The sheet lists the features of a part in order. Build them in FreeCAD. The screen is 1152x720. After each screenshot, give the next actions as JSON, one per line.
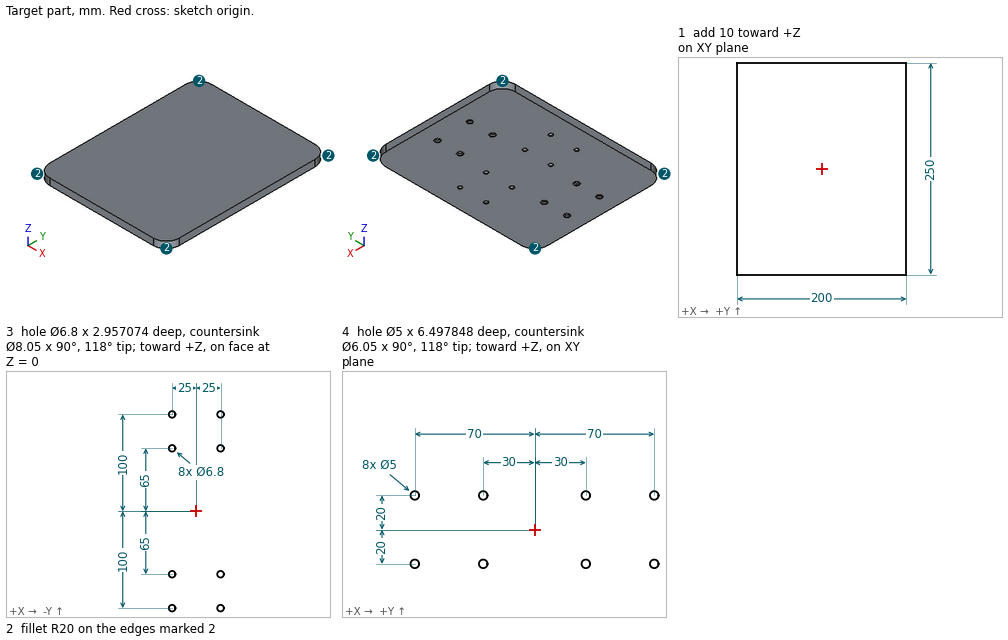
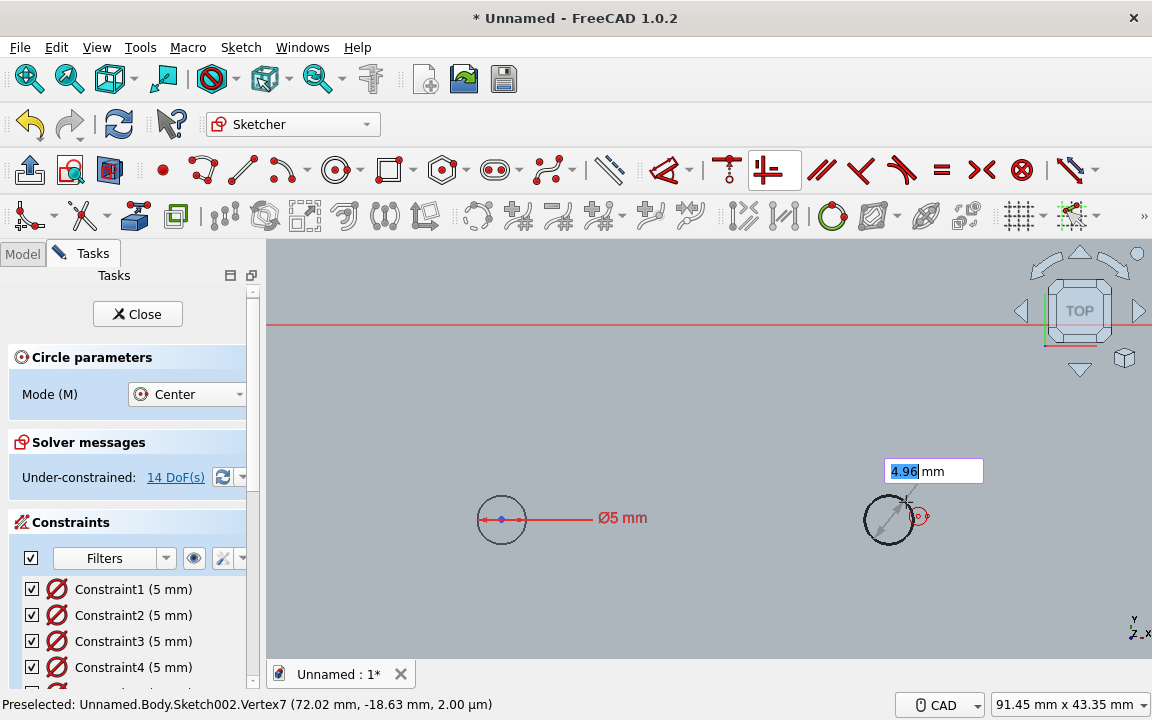
{"action": "type", "text": "5"}
{"action": "key", "text": "Return"}
{"action": "key", "text": "Escape"}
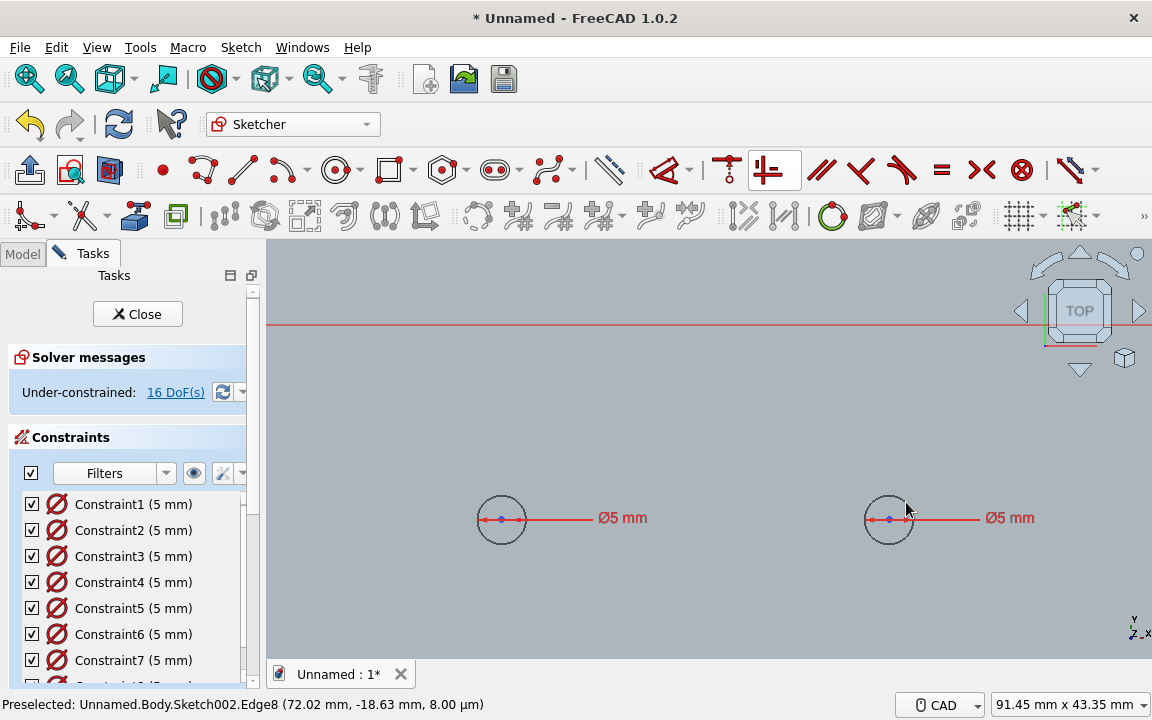
{"action": "scroll", "coordinate": [891, 521], "scroll_direction": "down", "scroll_amount": 5}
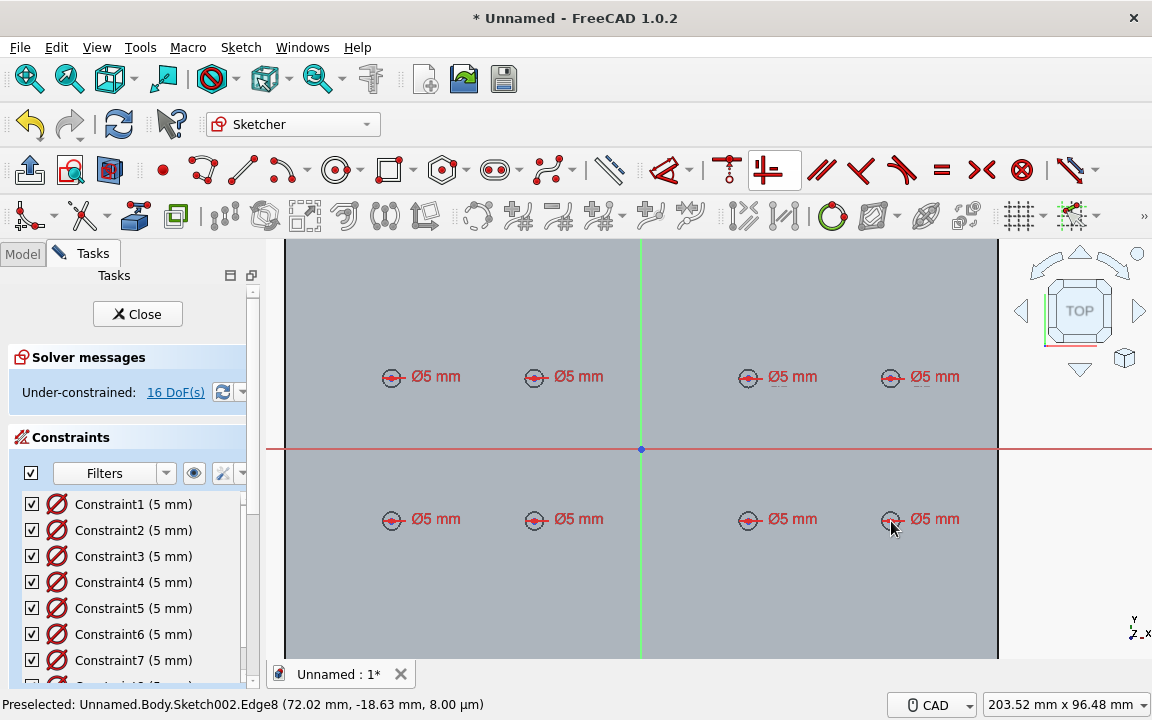
{"action": "left_click", "coordinate": [392, 378]}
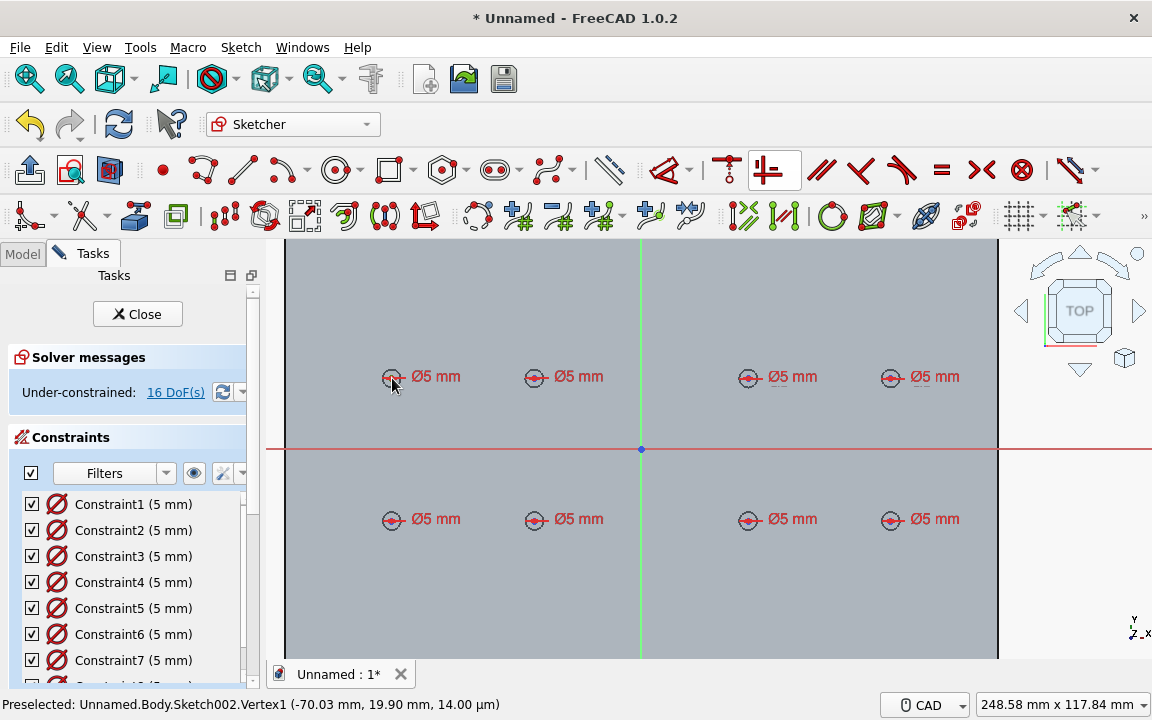
{"action": "left_click", "coordinate": [534, 378]}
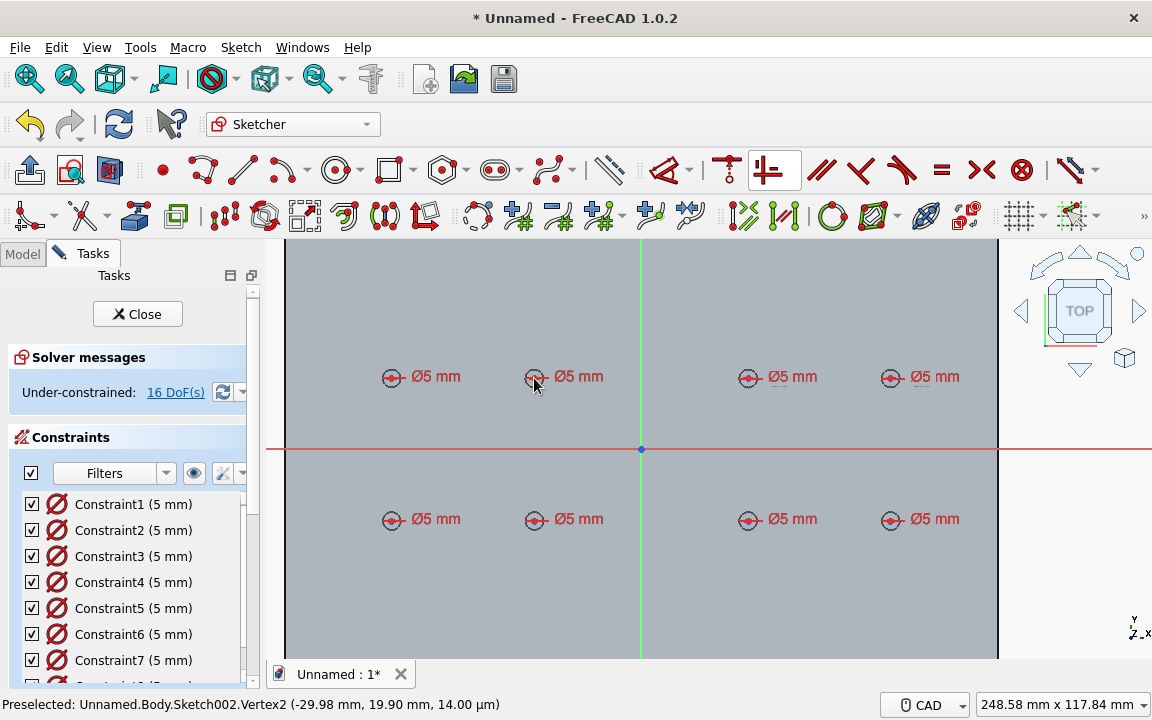
{"action": "key", "text": "h"}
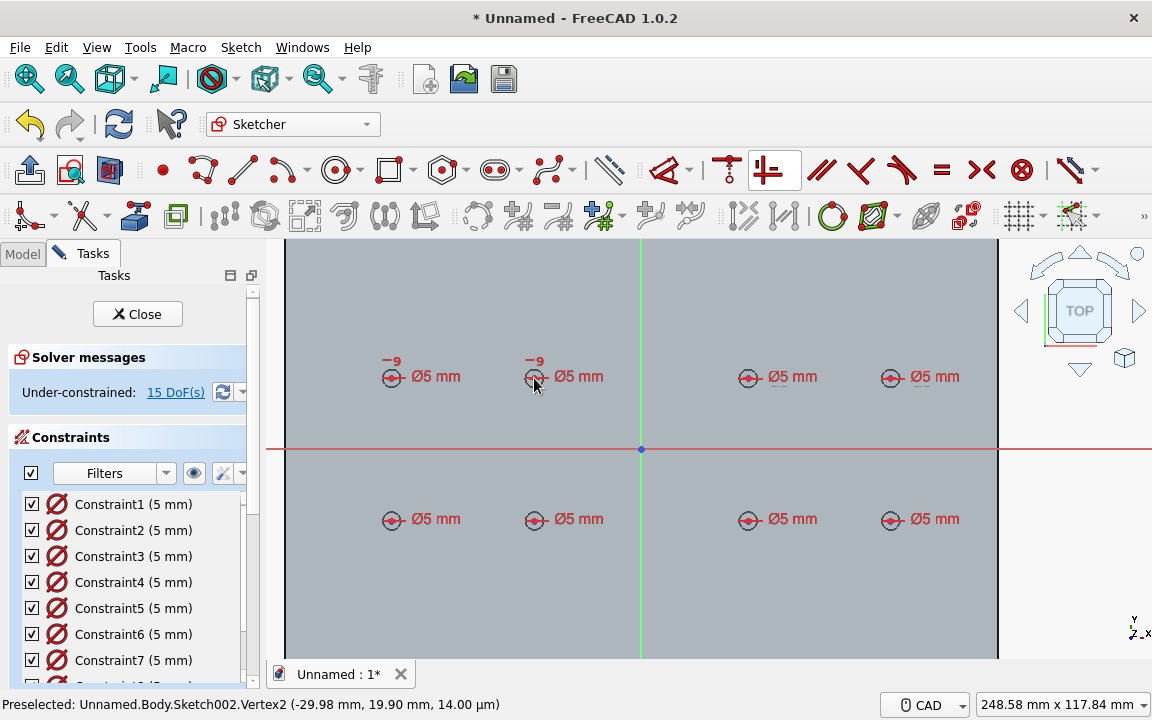
{"action": "left_click", "coordinate": [392, 378]}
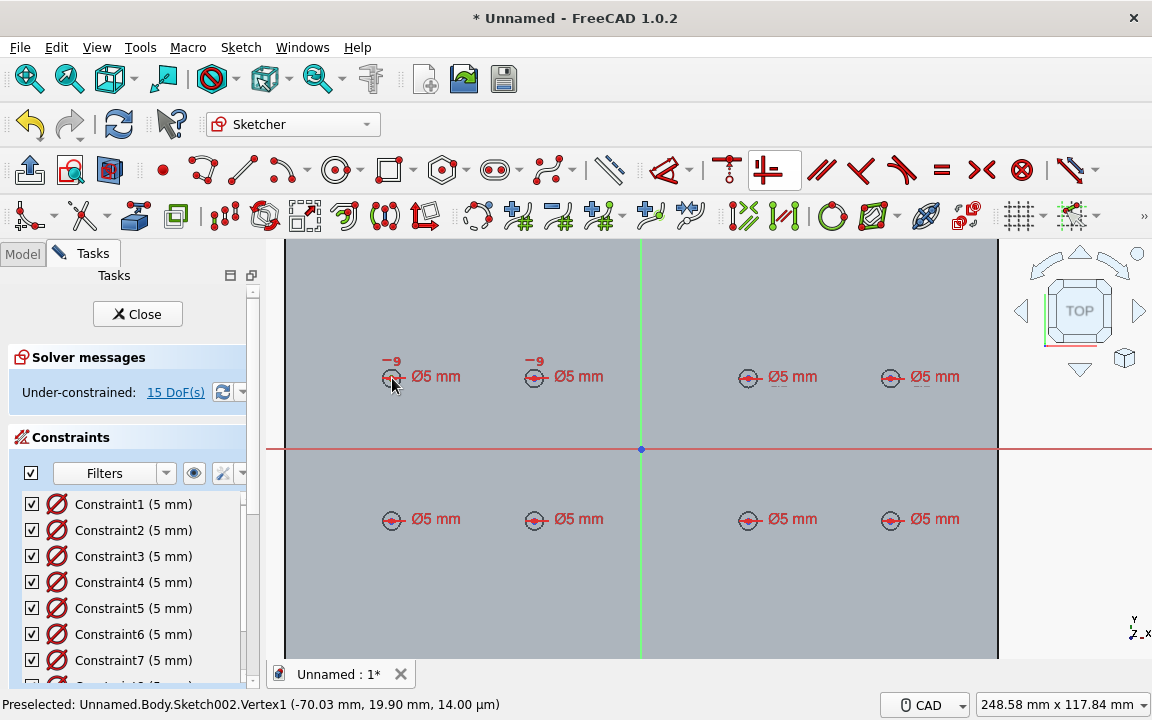
{"action": "left_click", "coordinate": [392, 521]}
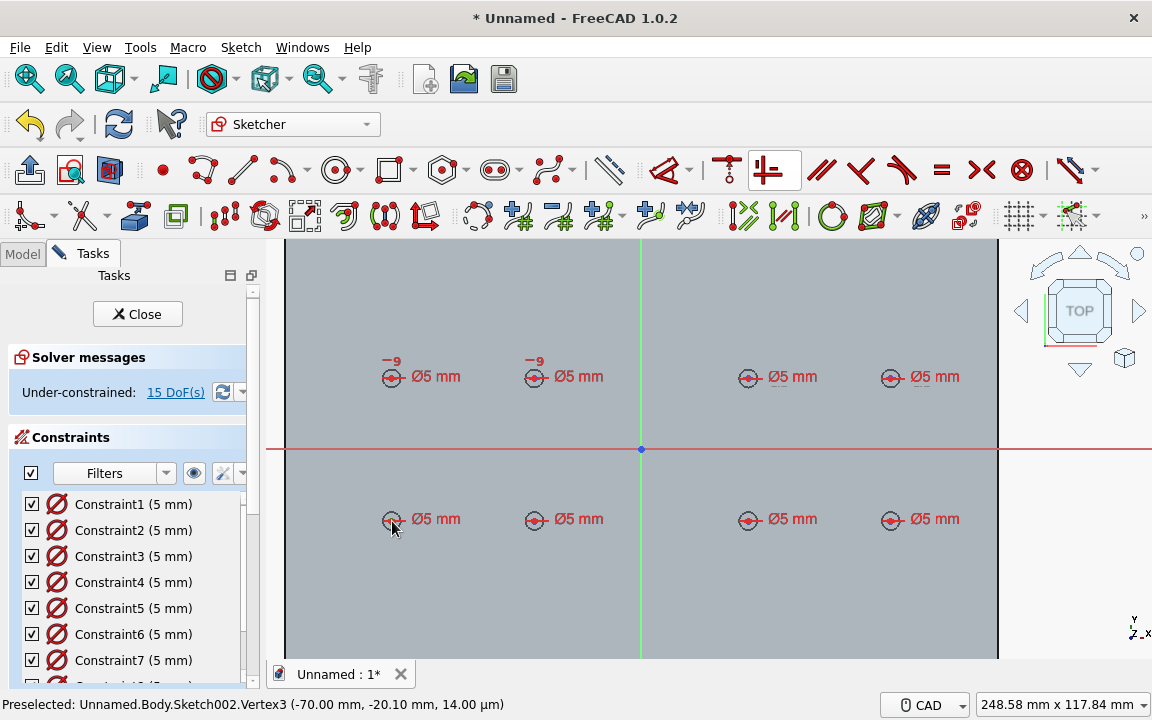
{"action": "key", "text": "v"}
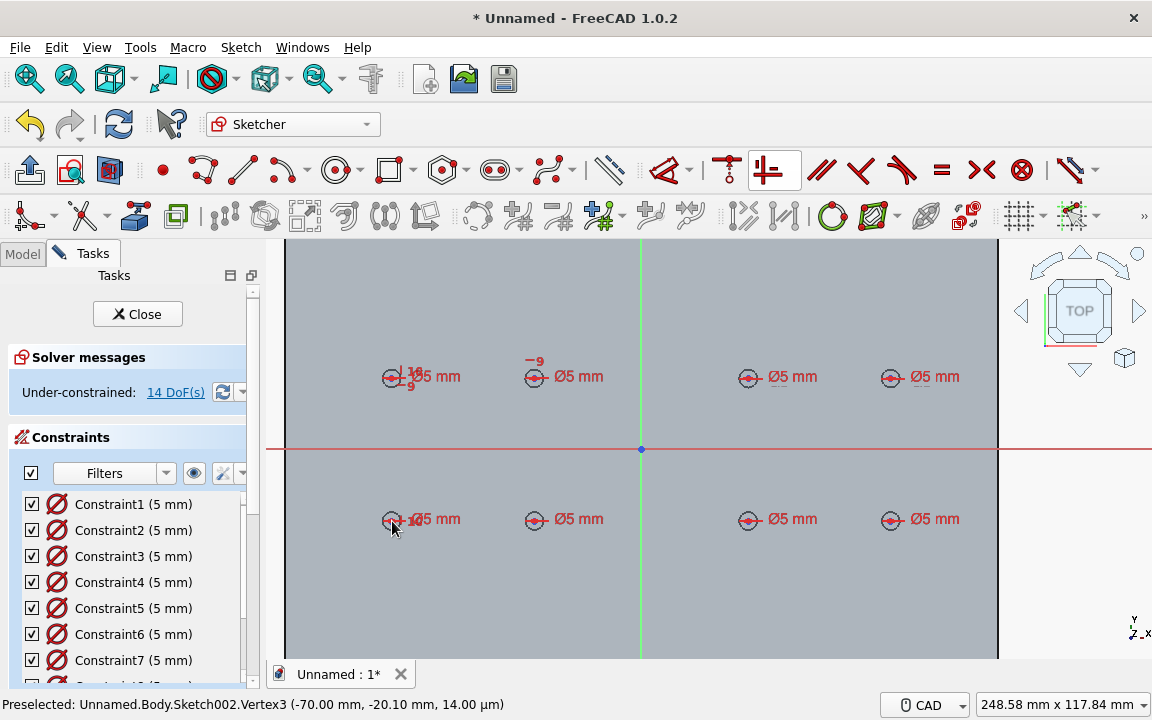
{"action": "left_click", "coordinate": [534, 378]}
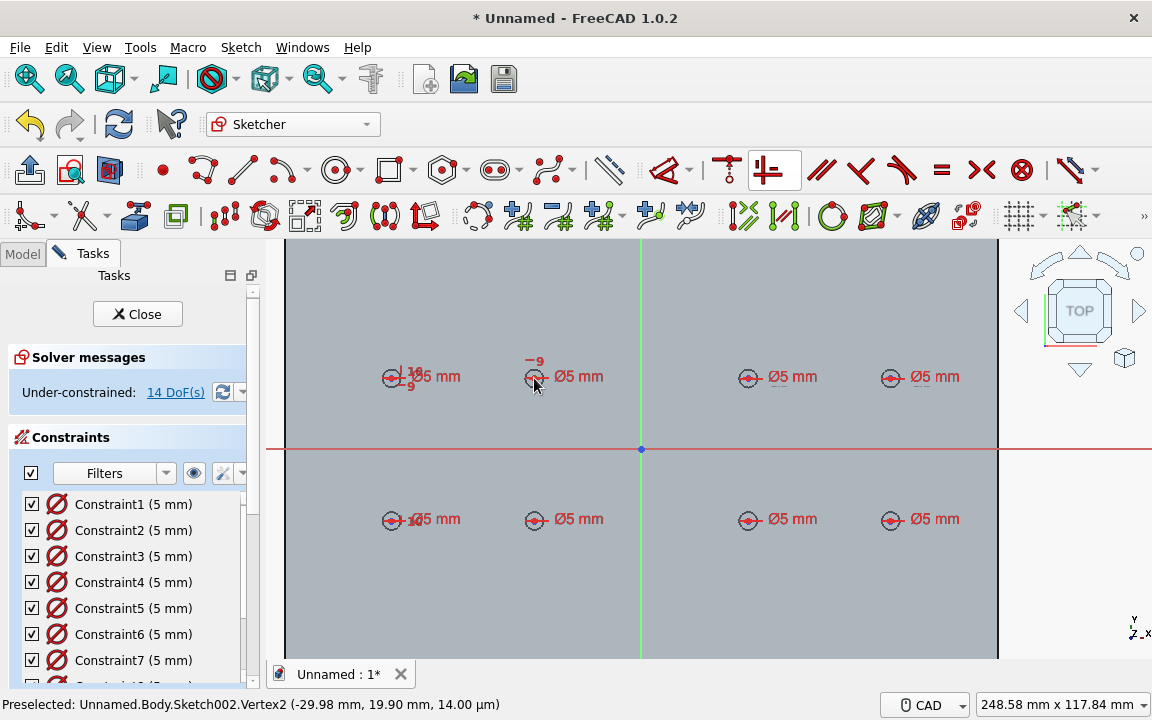
{"action": "left_click", "coordinate": [534, 521]}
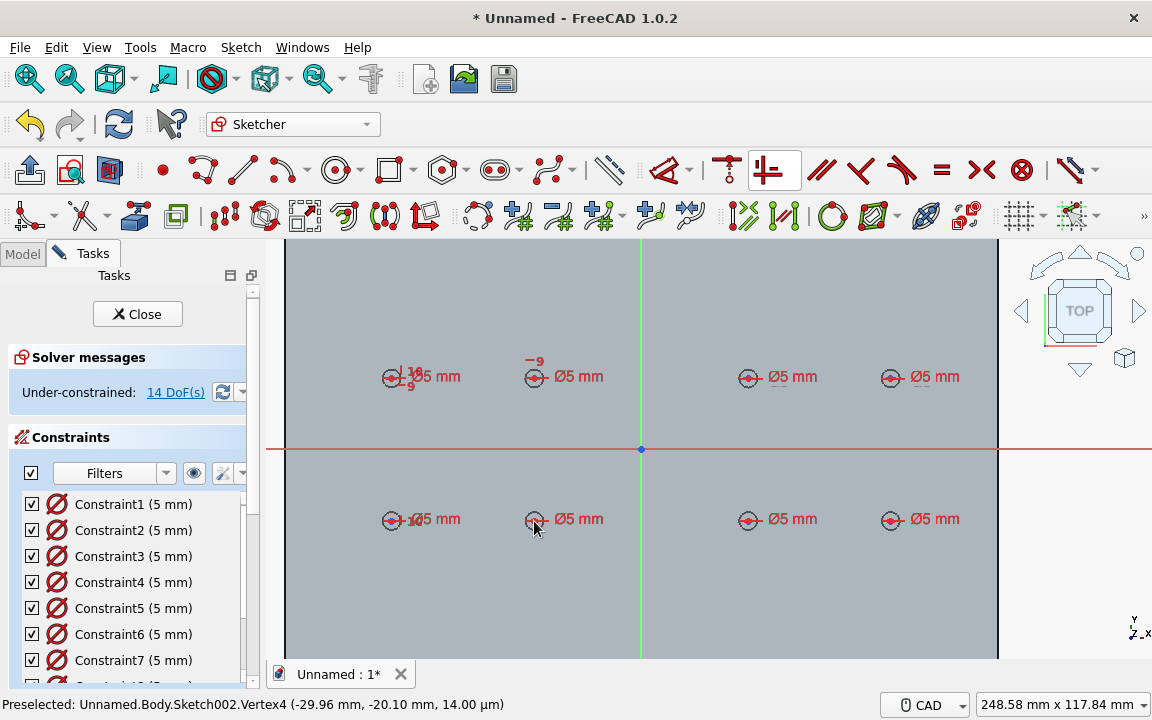
{"action": "left_click", "coordinate": [796, 170]}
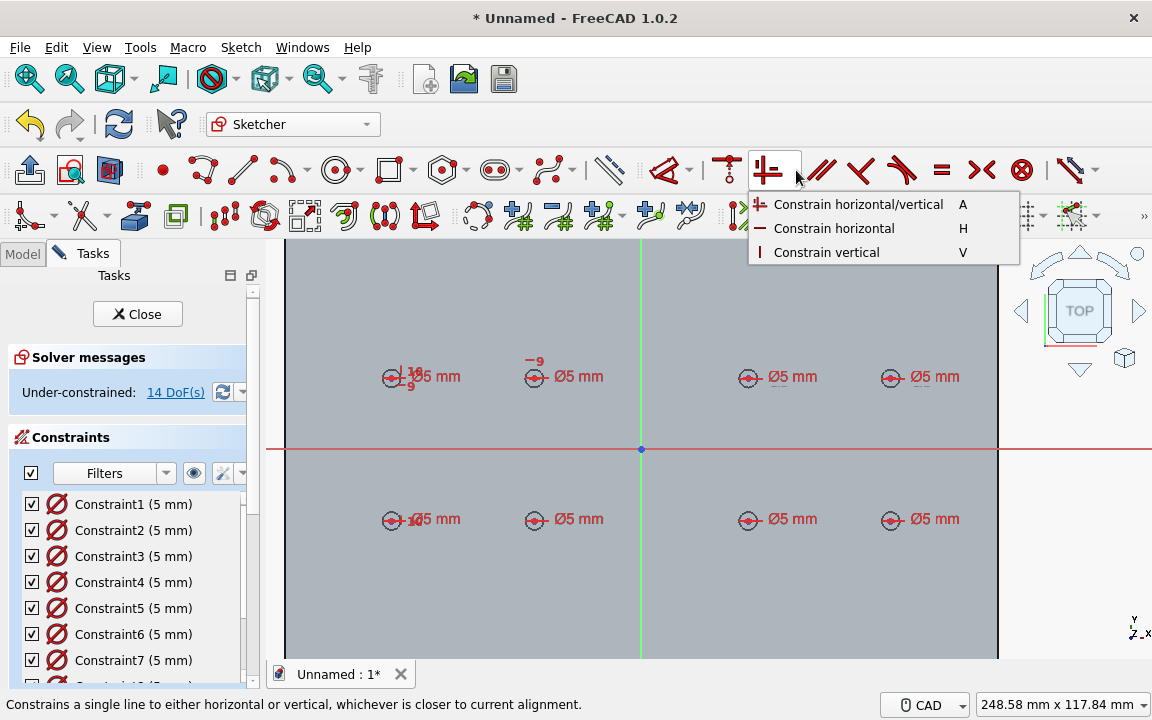
{"action": "left_click", "coordinate": [884, 252]}